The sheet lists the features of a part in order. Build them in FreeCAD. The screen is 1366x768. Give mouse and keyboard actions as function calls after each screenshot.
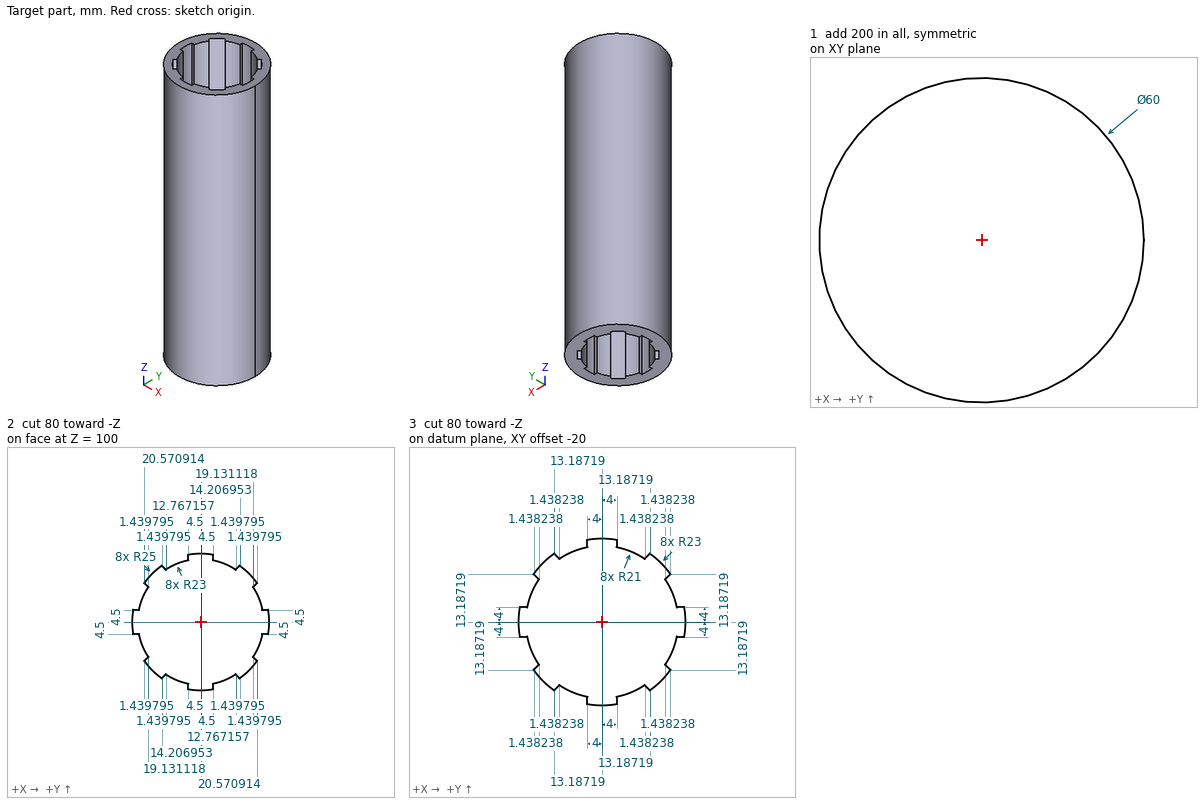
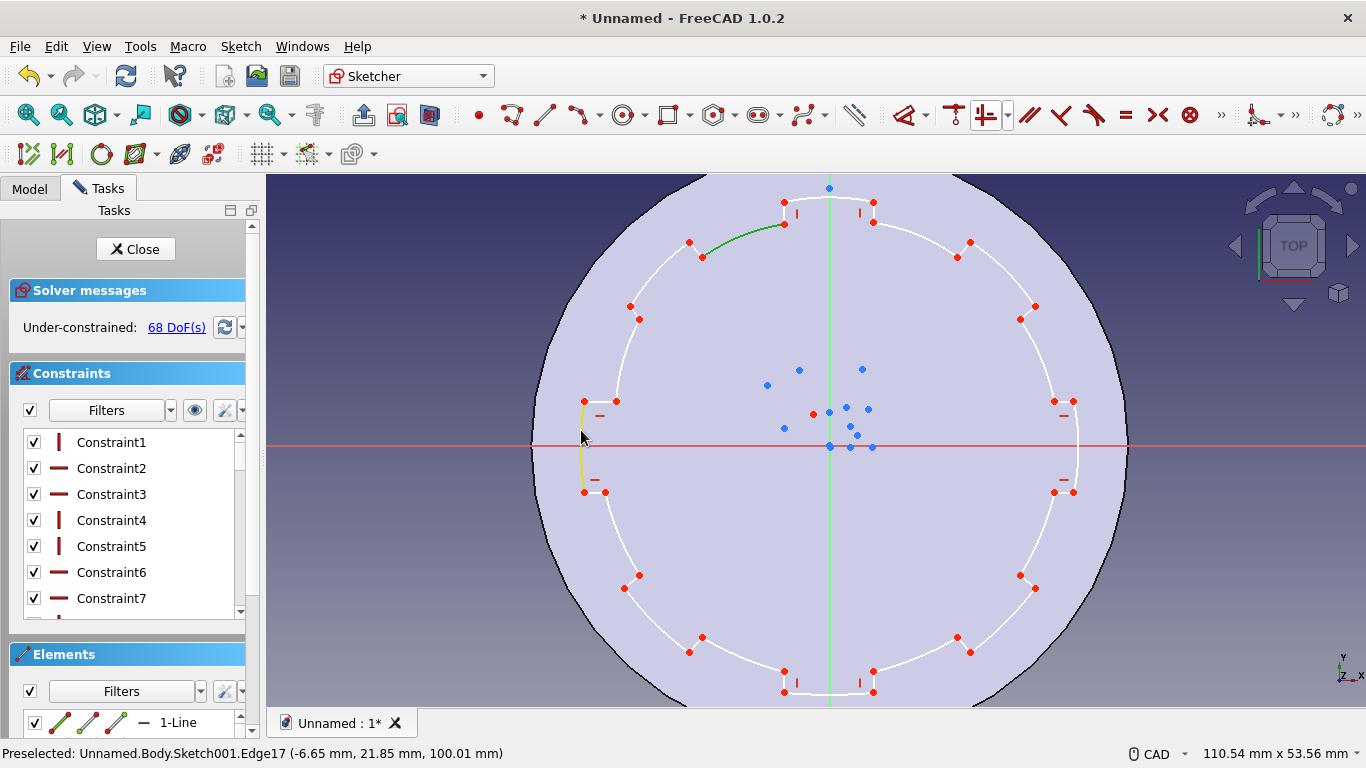
click(582, 429)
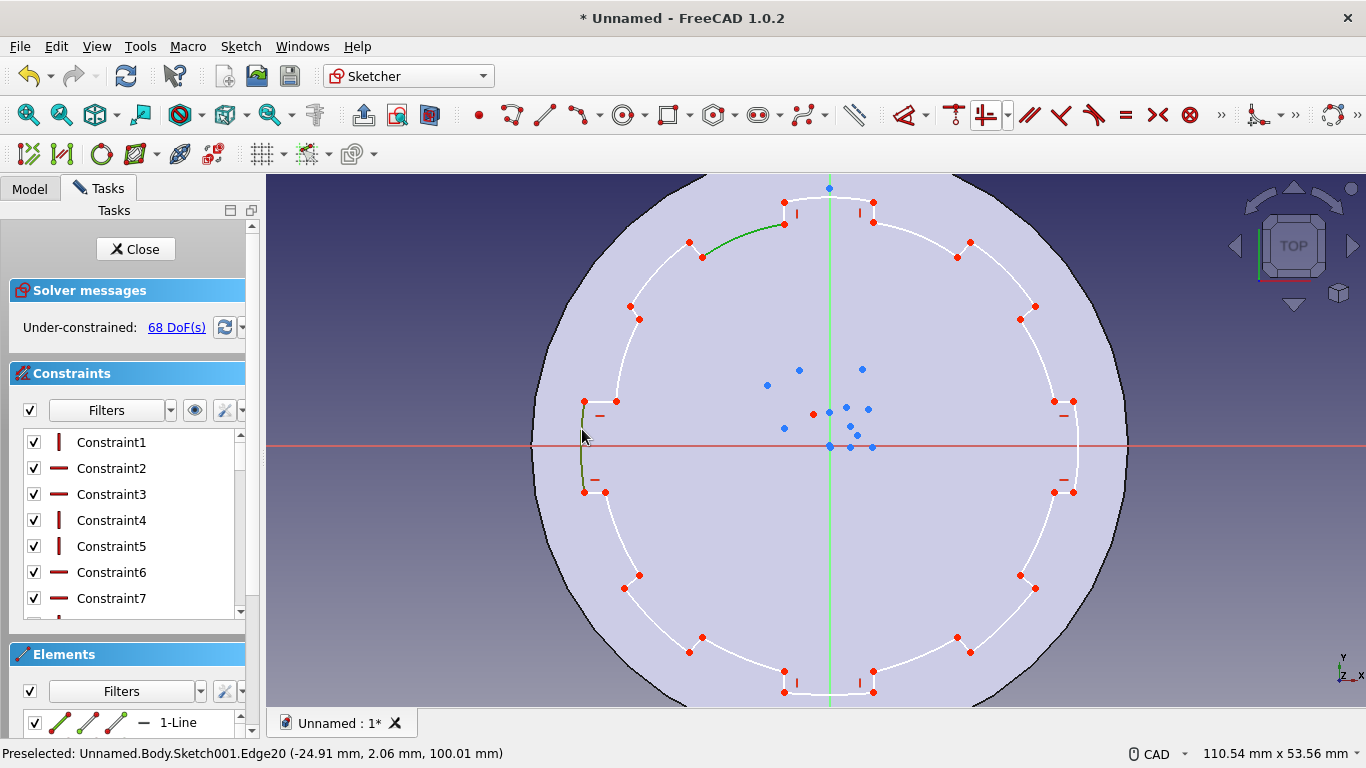
click(954, 116)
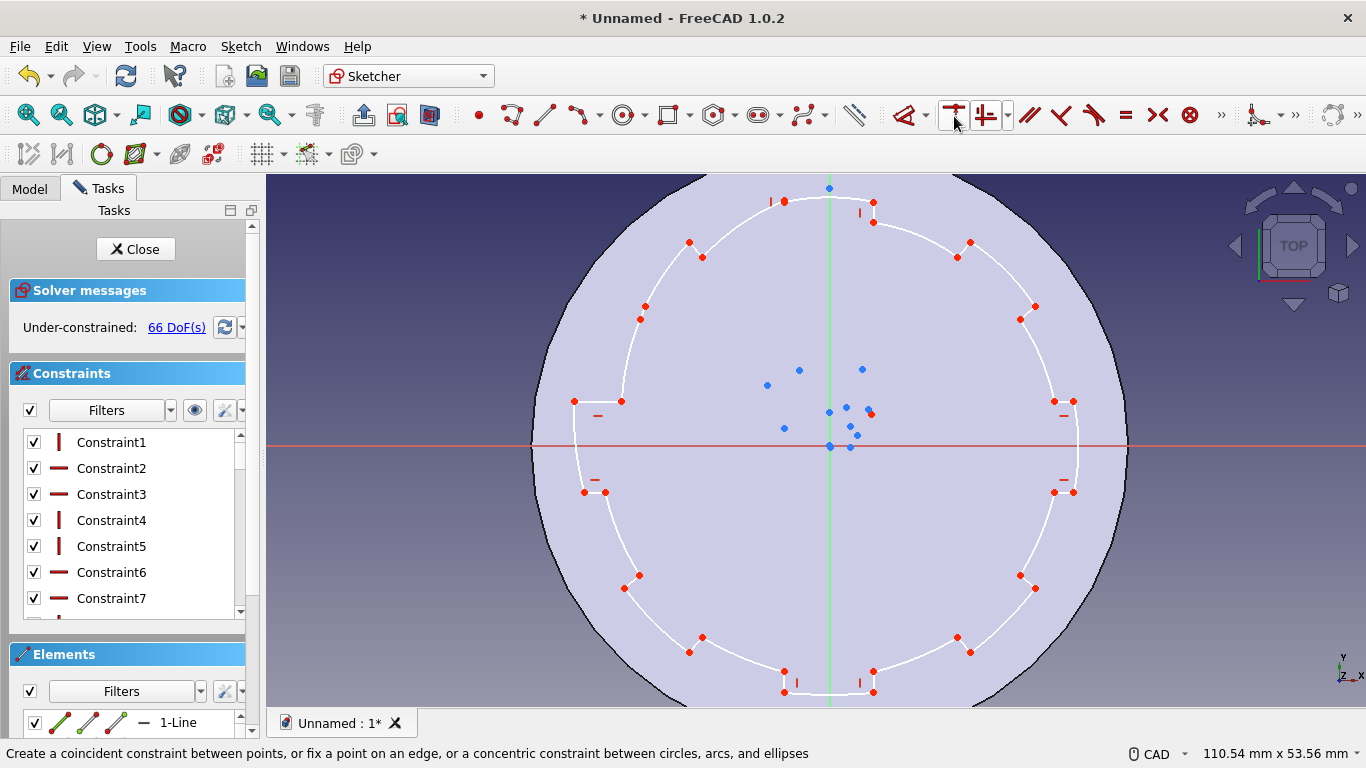
click(758, 214)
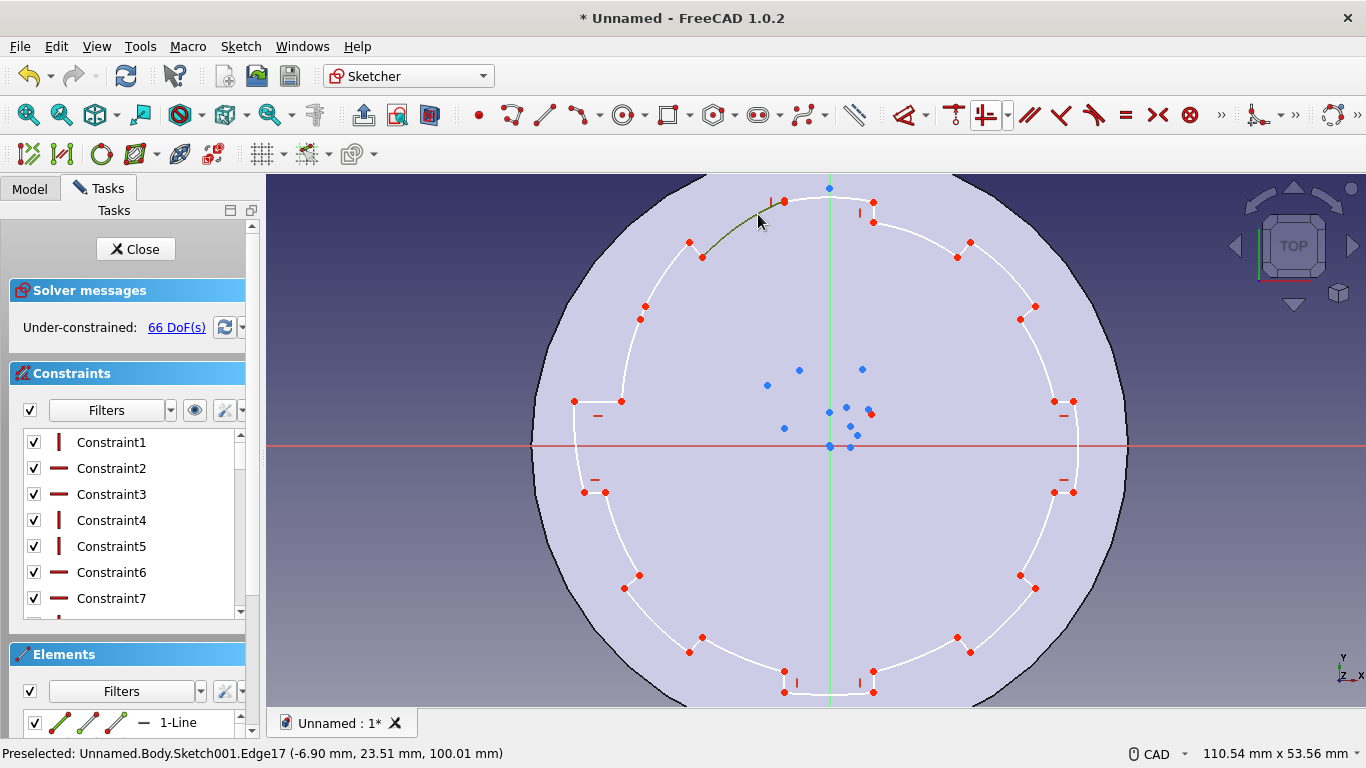
click(613, 519)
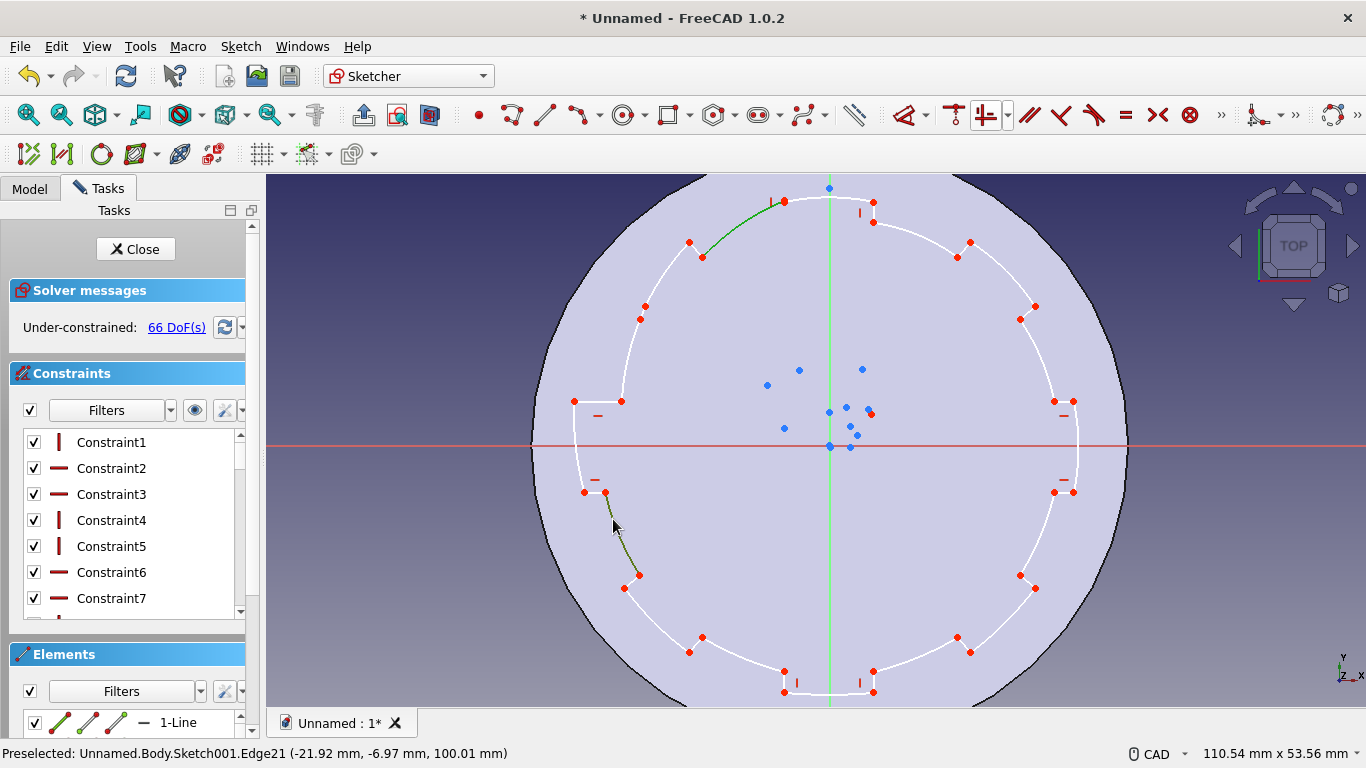
click(954, 116)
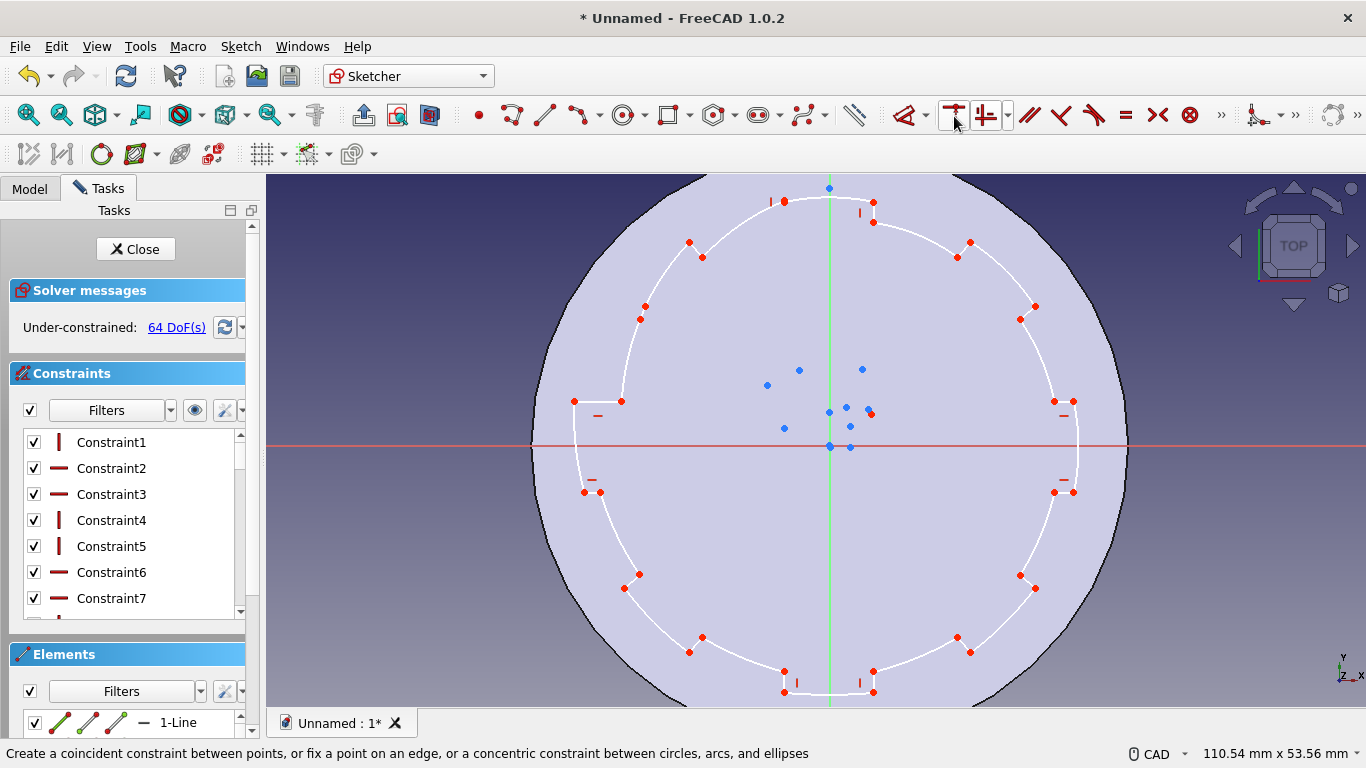
click(758, 214)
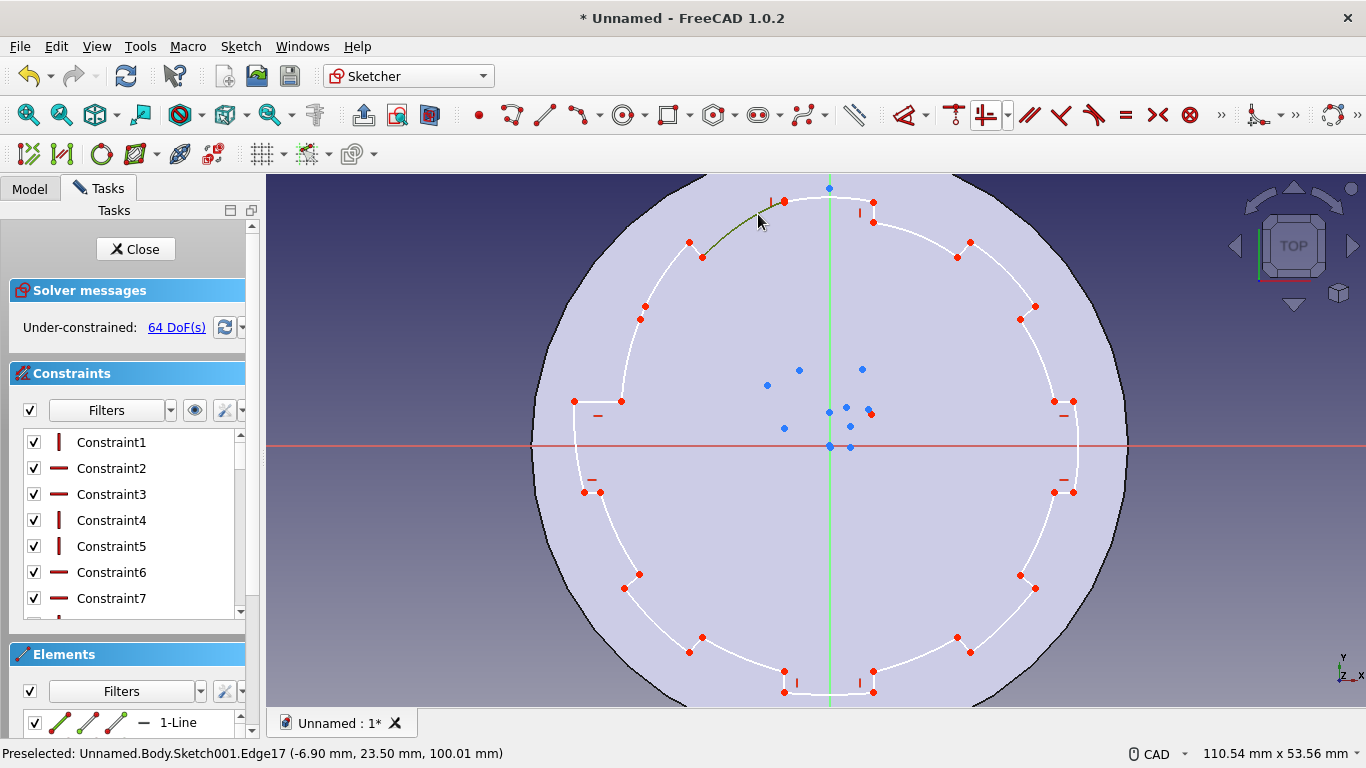
click(642, 610)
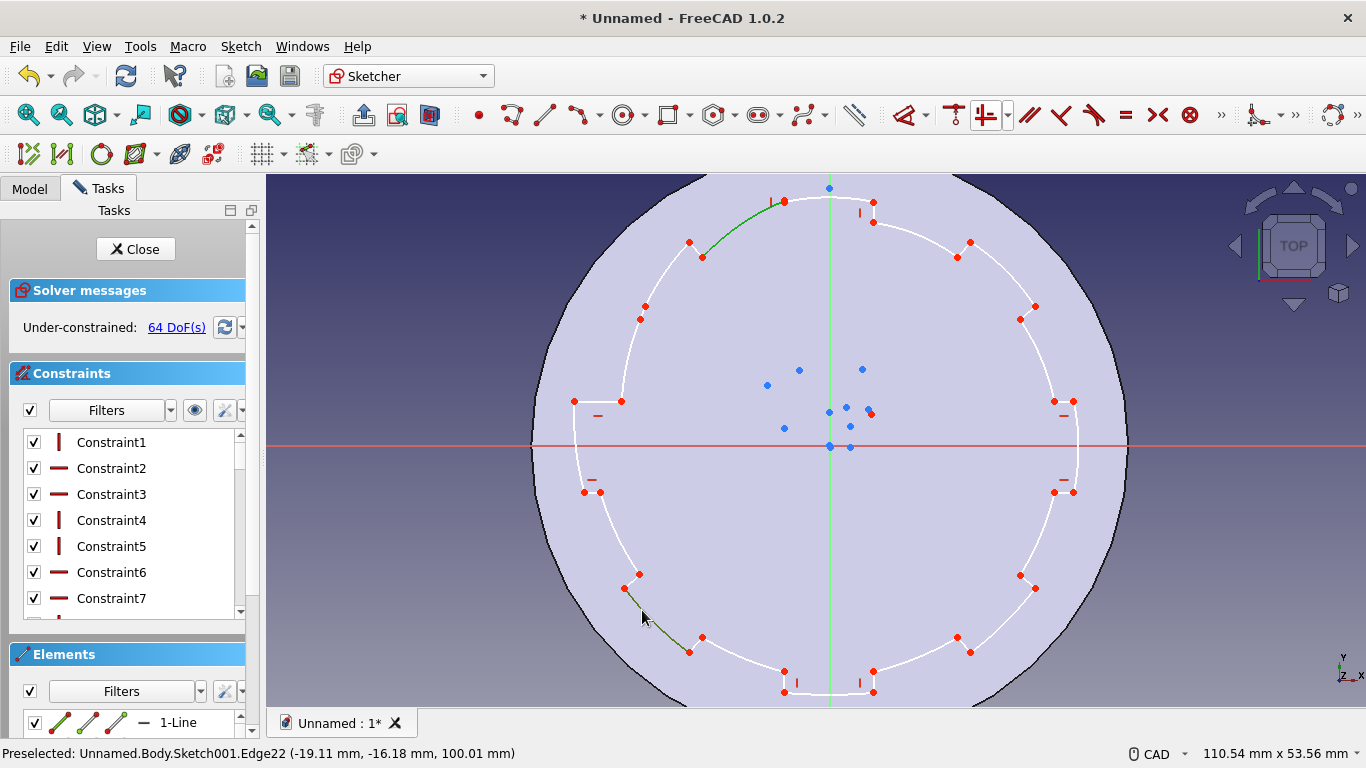
click(954, 116)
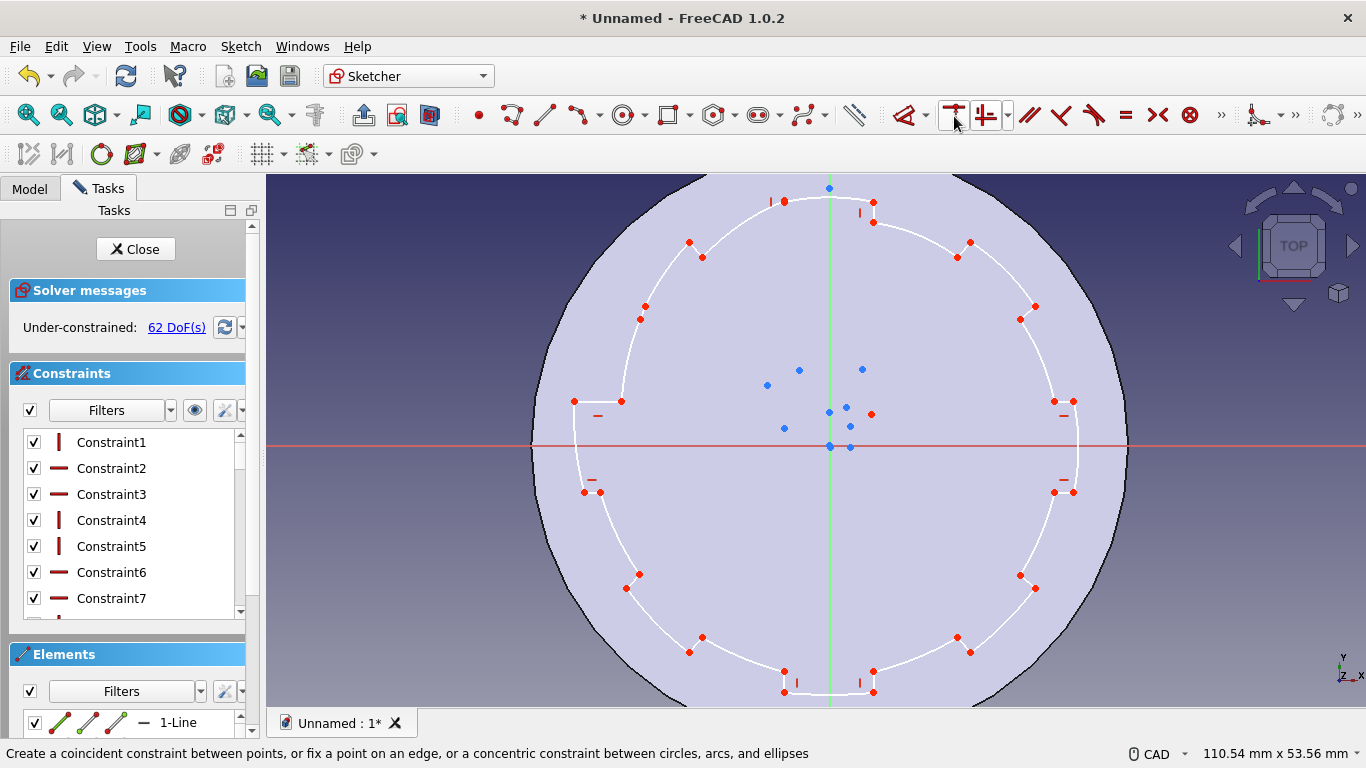
click(758, 214)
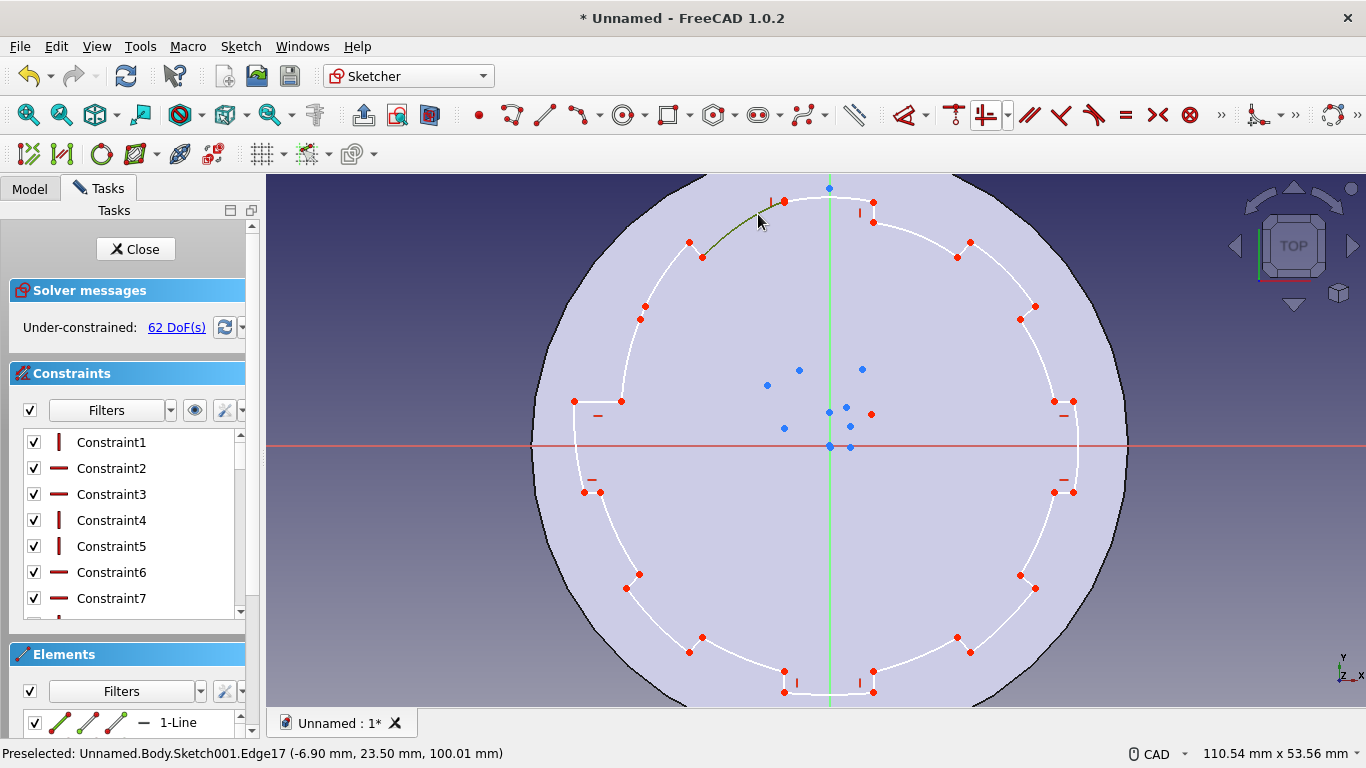
click(726, 650)